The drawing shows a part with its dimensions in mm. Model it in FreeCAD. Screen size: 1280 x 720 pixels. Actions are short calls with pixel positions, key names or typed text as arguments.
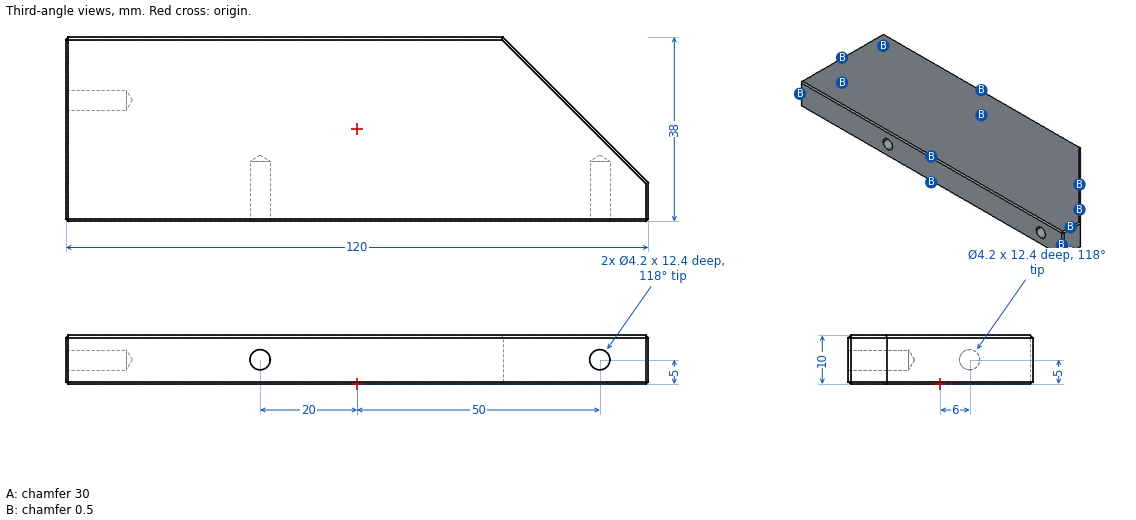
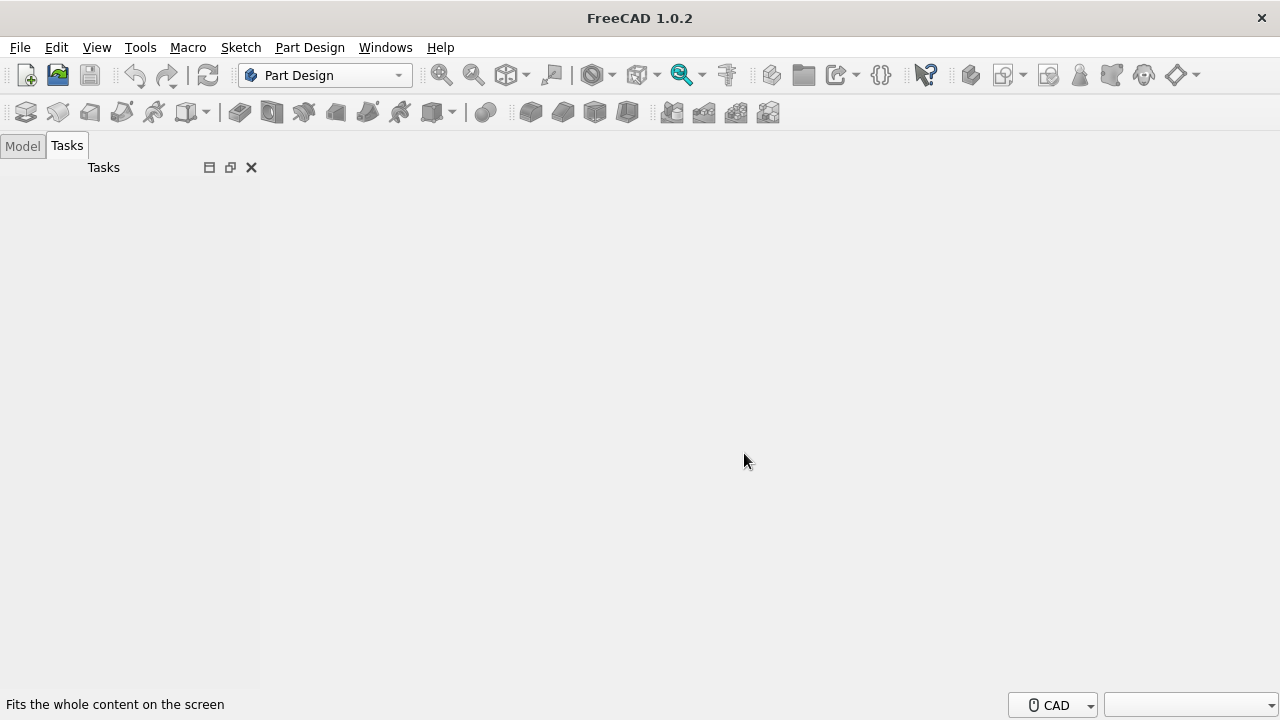
click(26, 76)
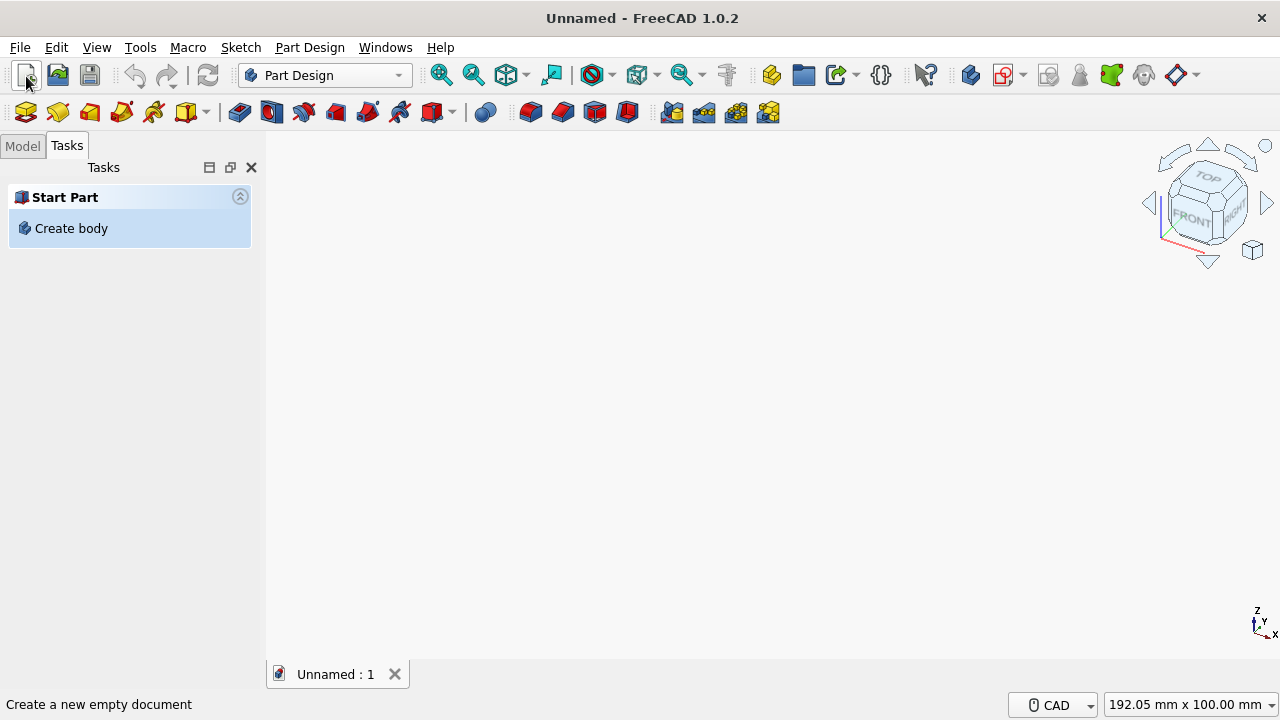
click(1004, 76)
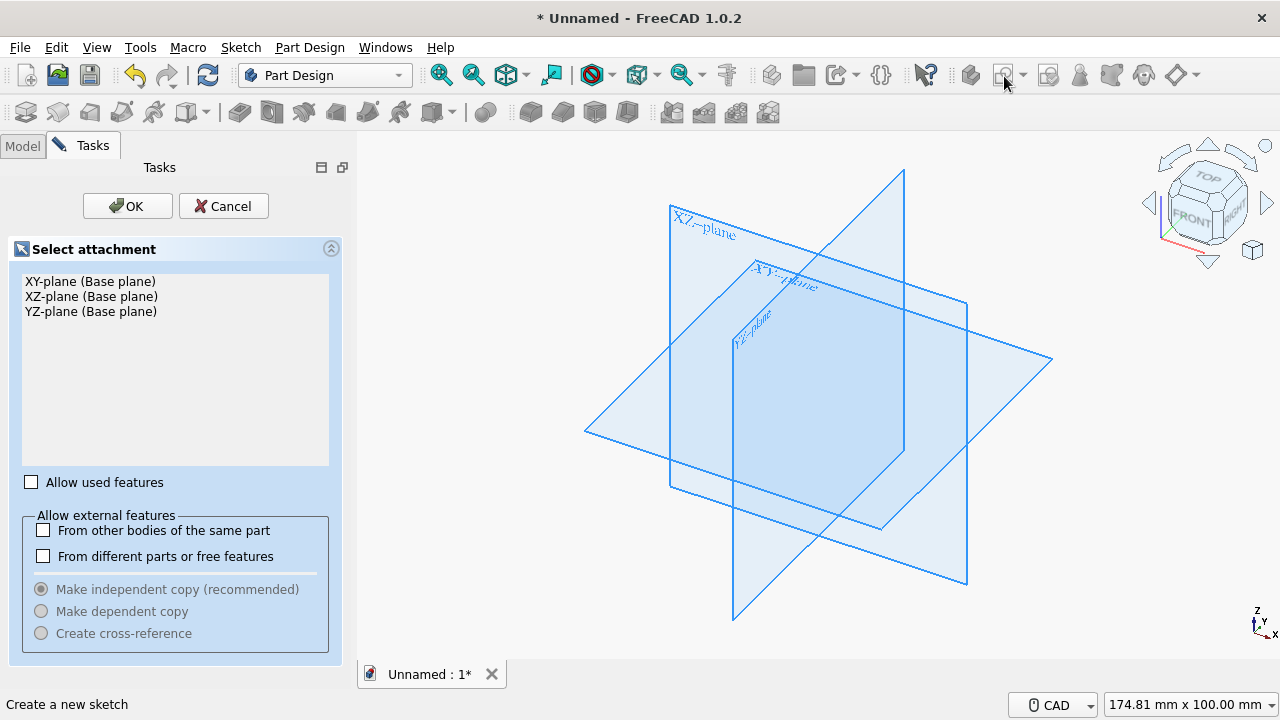
click(82, 282)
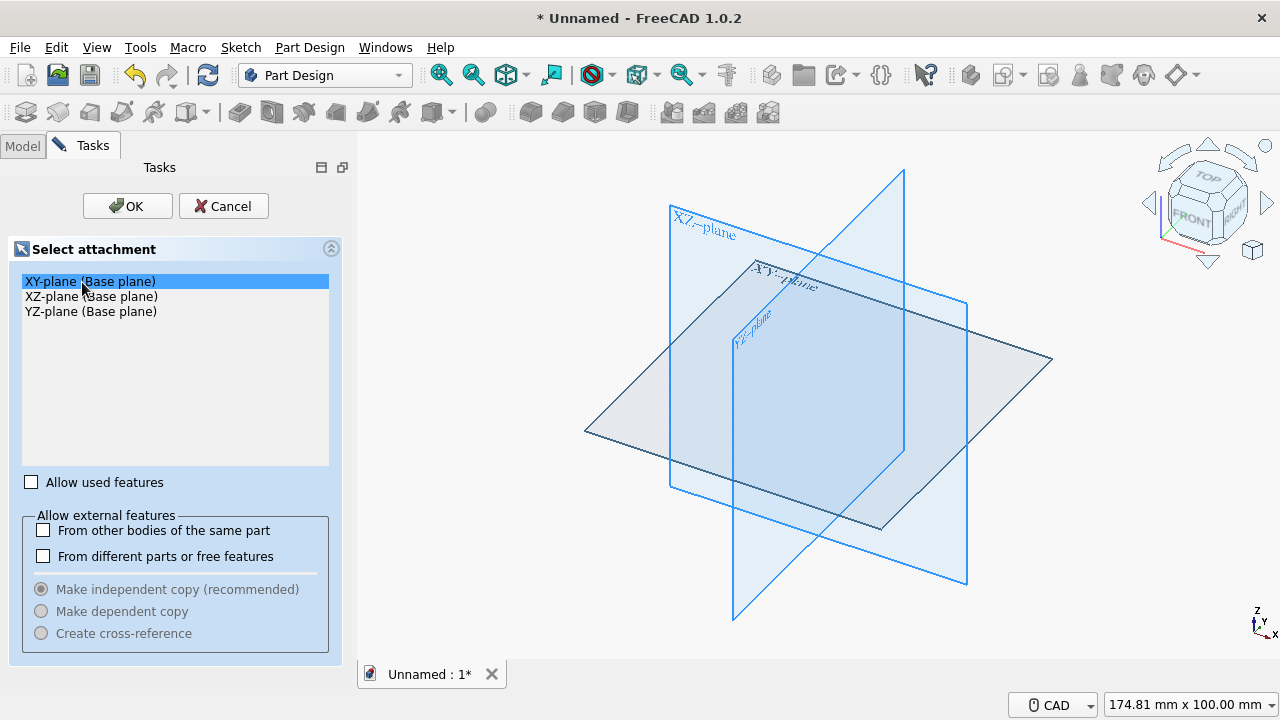
click(128, 206)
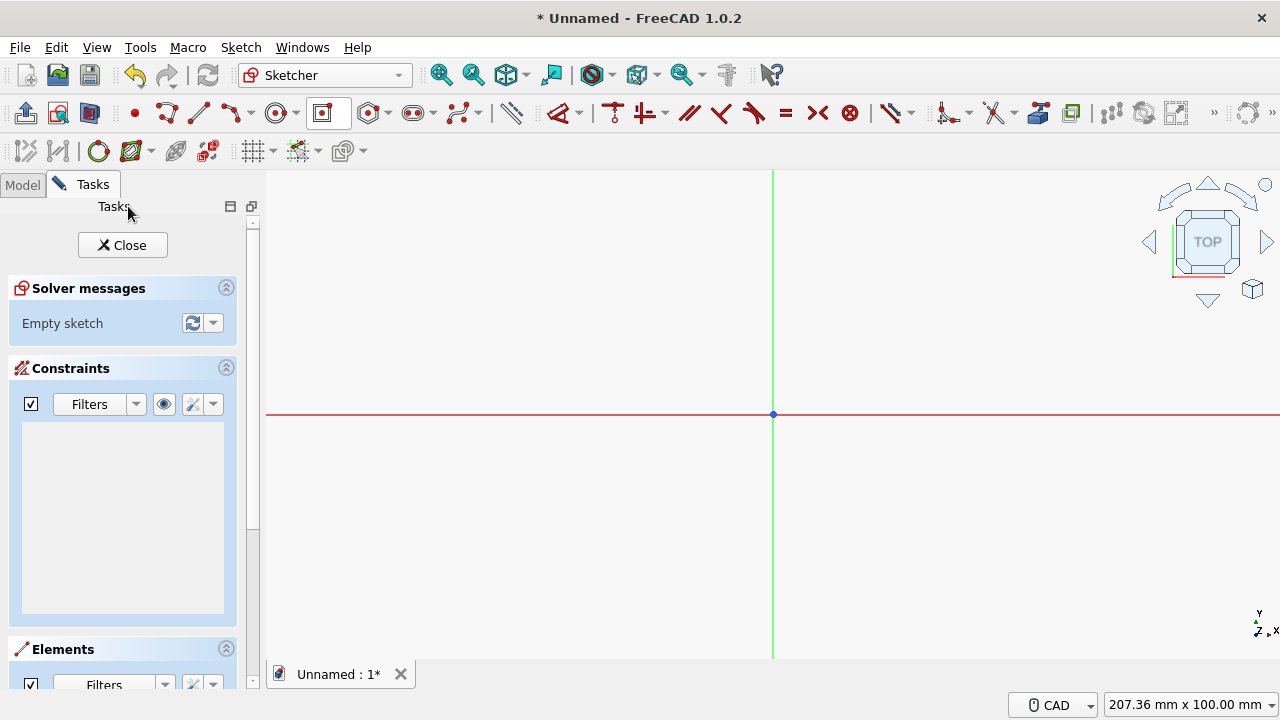
click(322, 114)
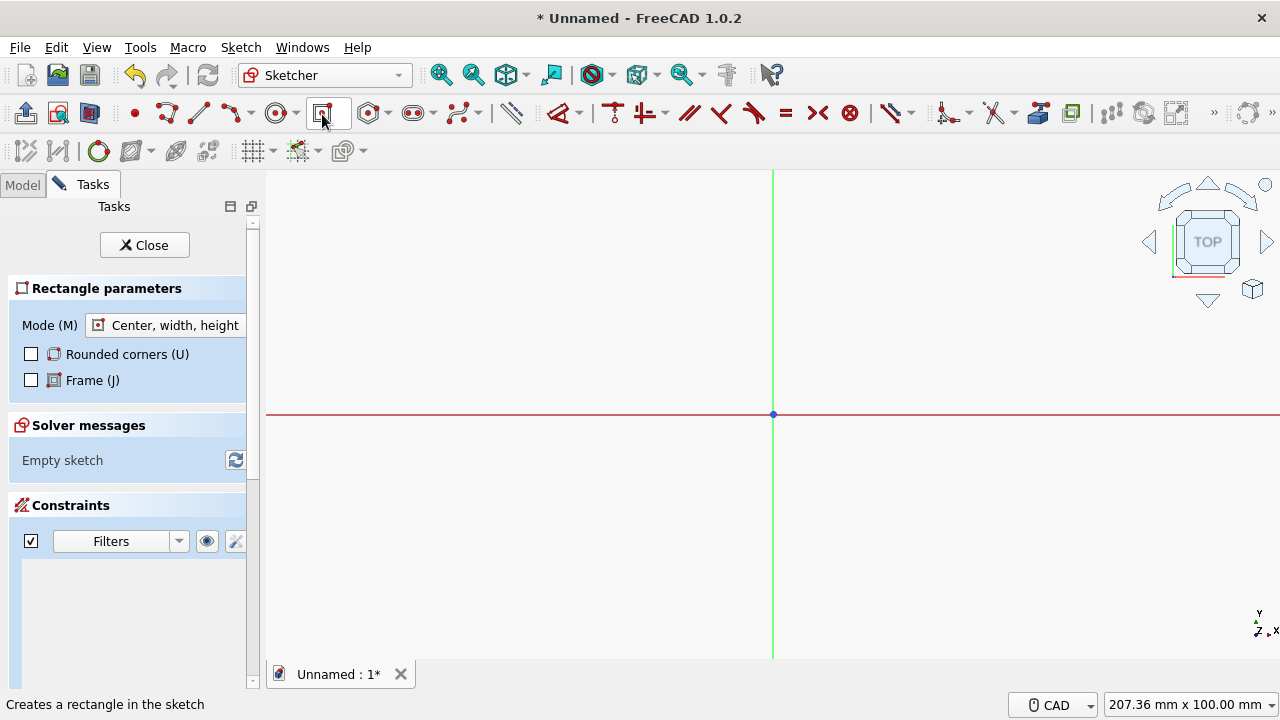
click(773, 414)
click(1066, 322)
key(Escape)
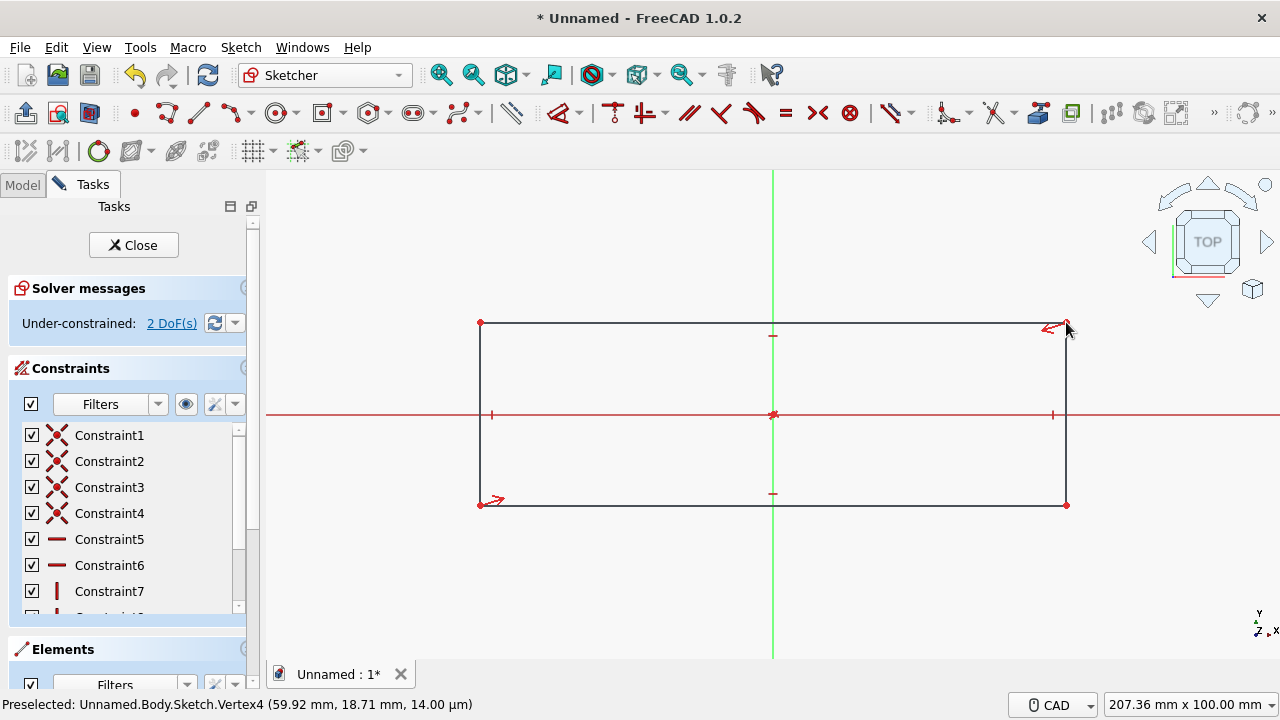
click(1066, 451)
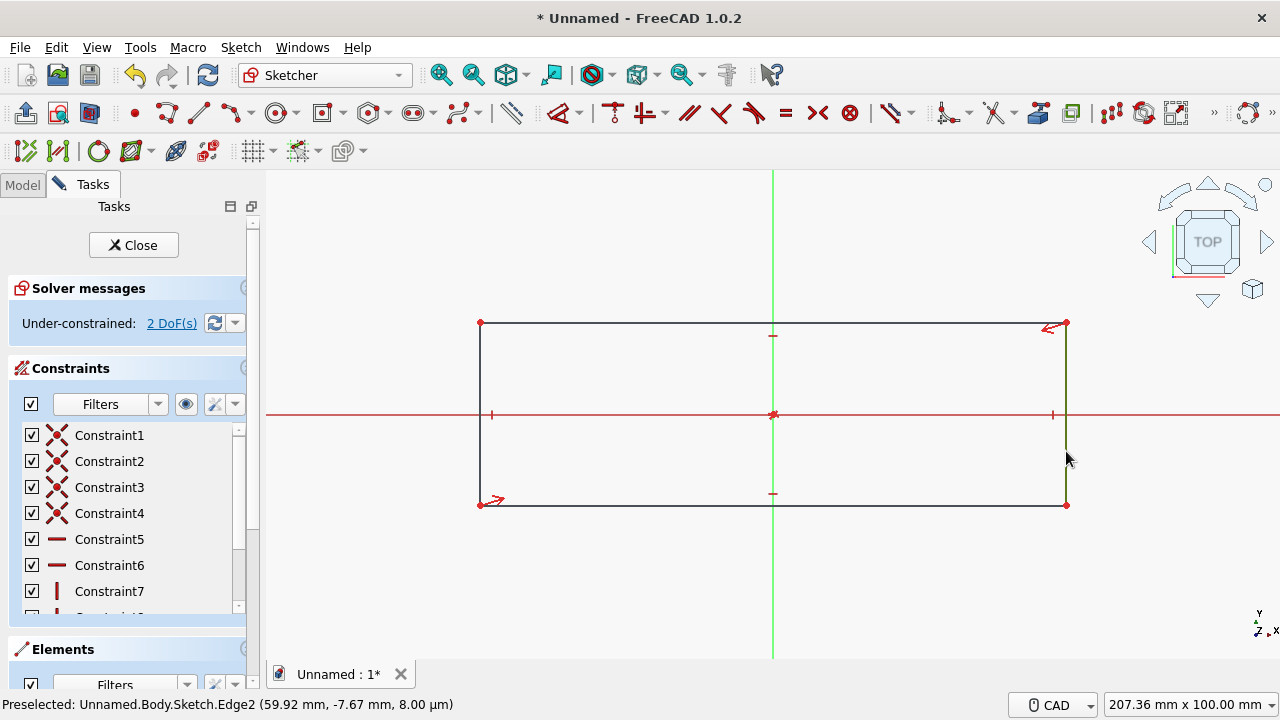
click(582, 114)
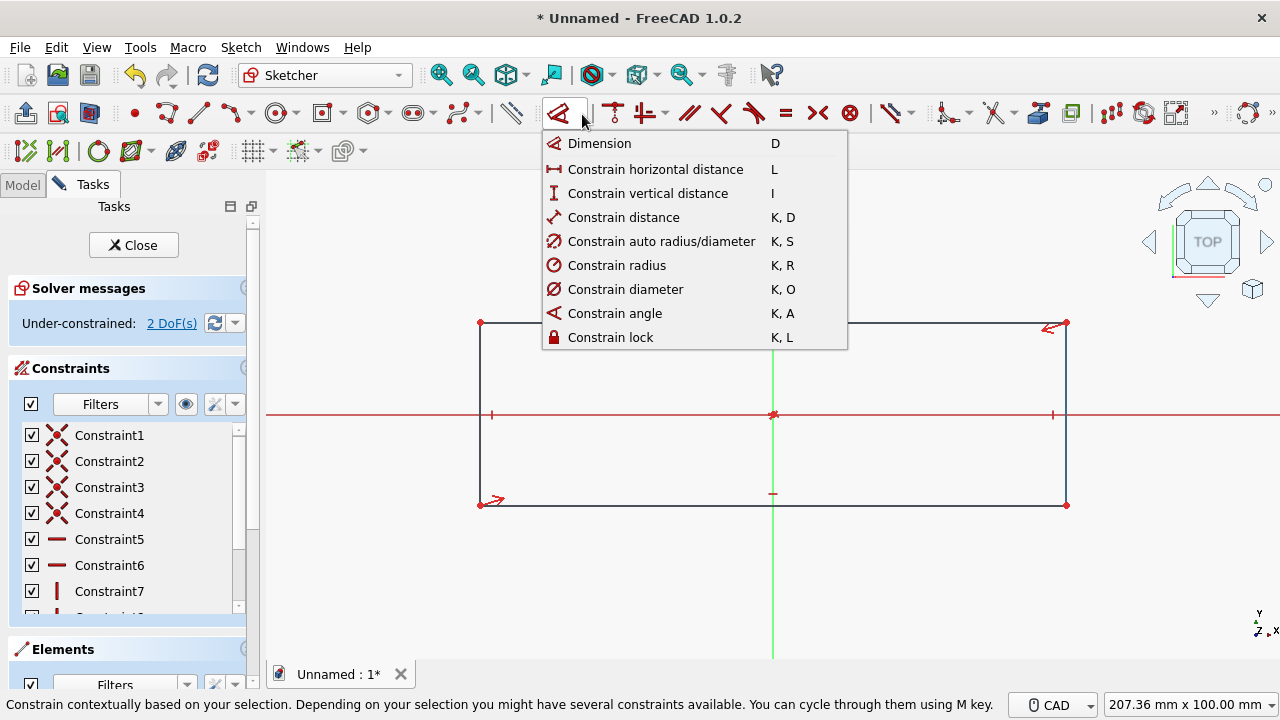
click(695, 193)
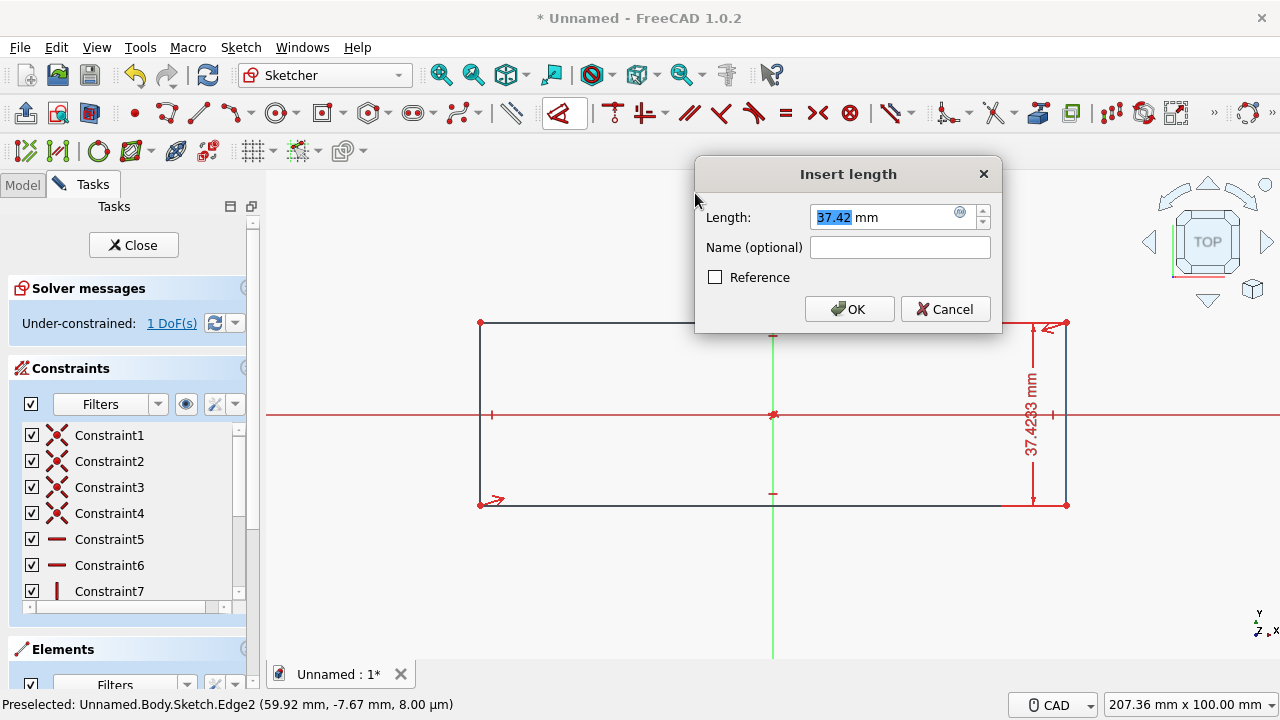
text(38)
key(Return)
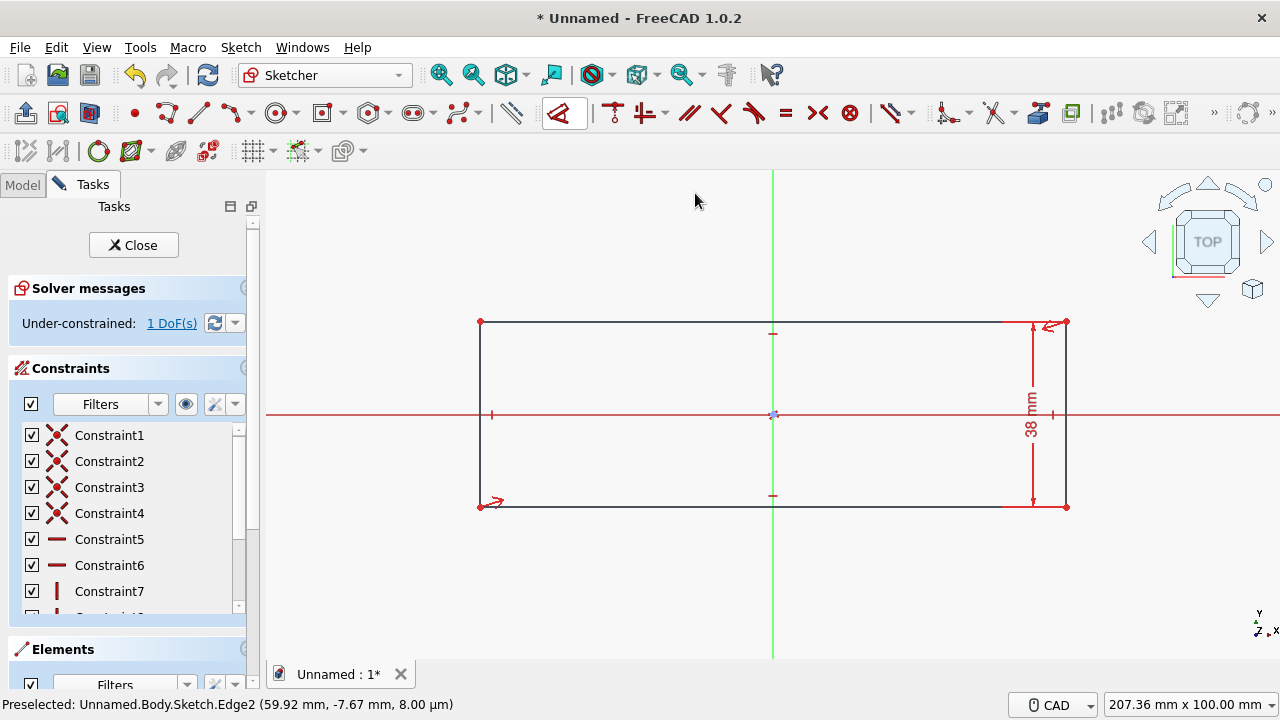
click(656, 507)